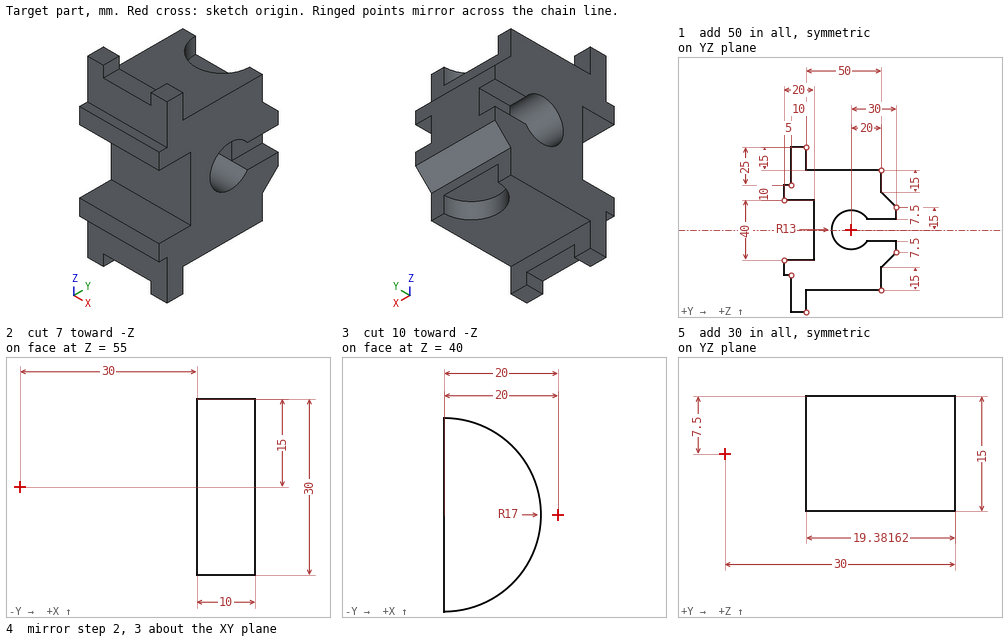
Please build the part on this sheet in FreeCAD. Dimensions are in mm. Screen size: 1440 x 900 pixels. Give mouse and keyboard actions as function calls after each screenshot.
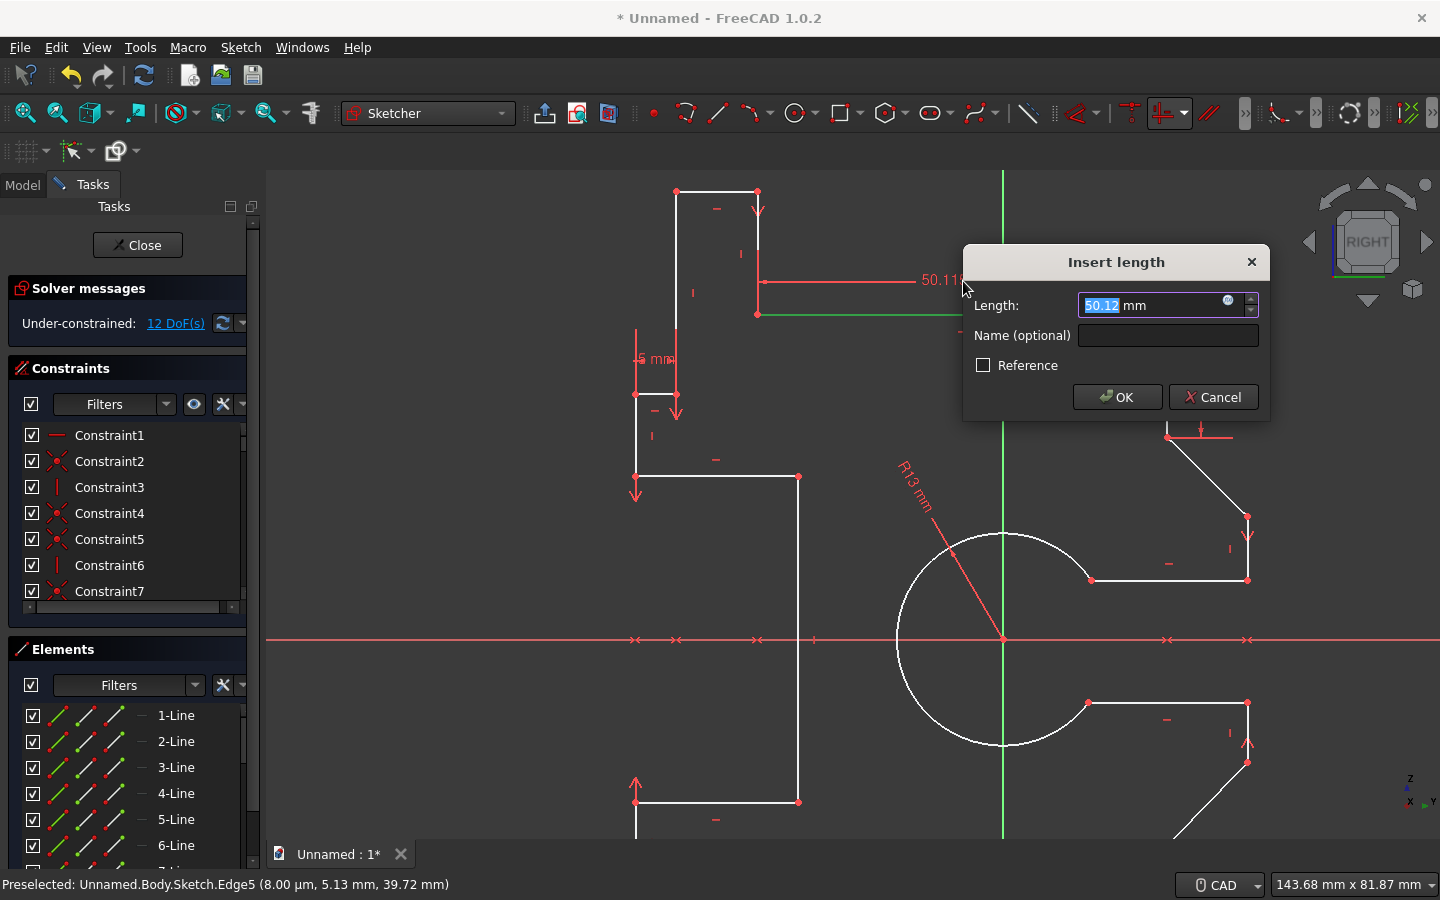
text(50)
key(Return)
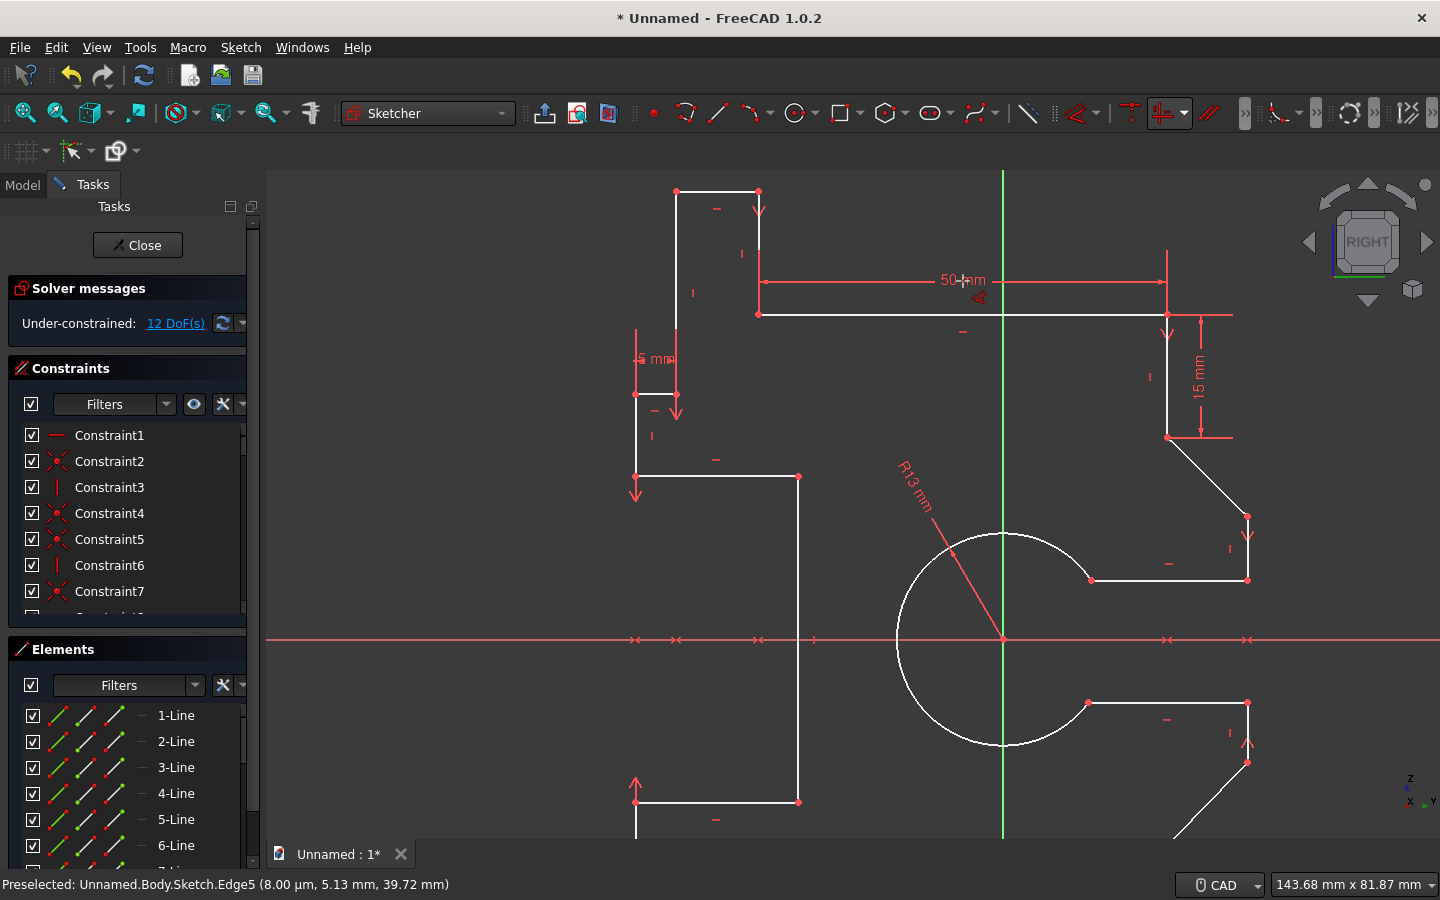
click(759, 278)
click(725, 256)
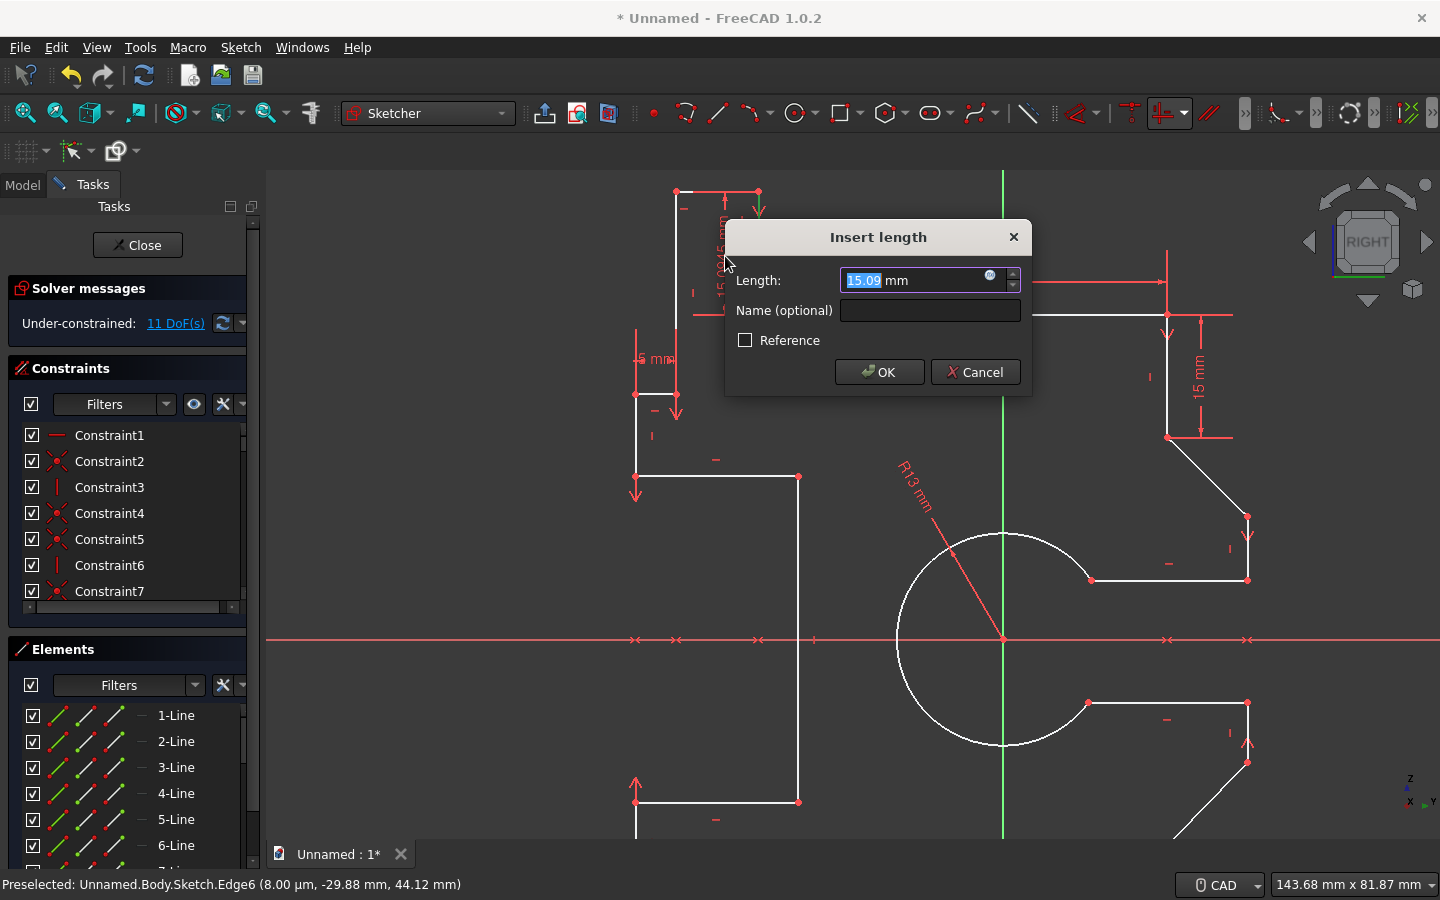
text(15)
key(Return)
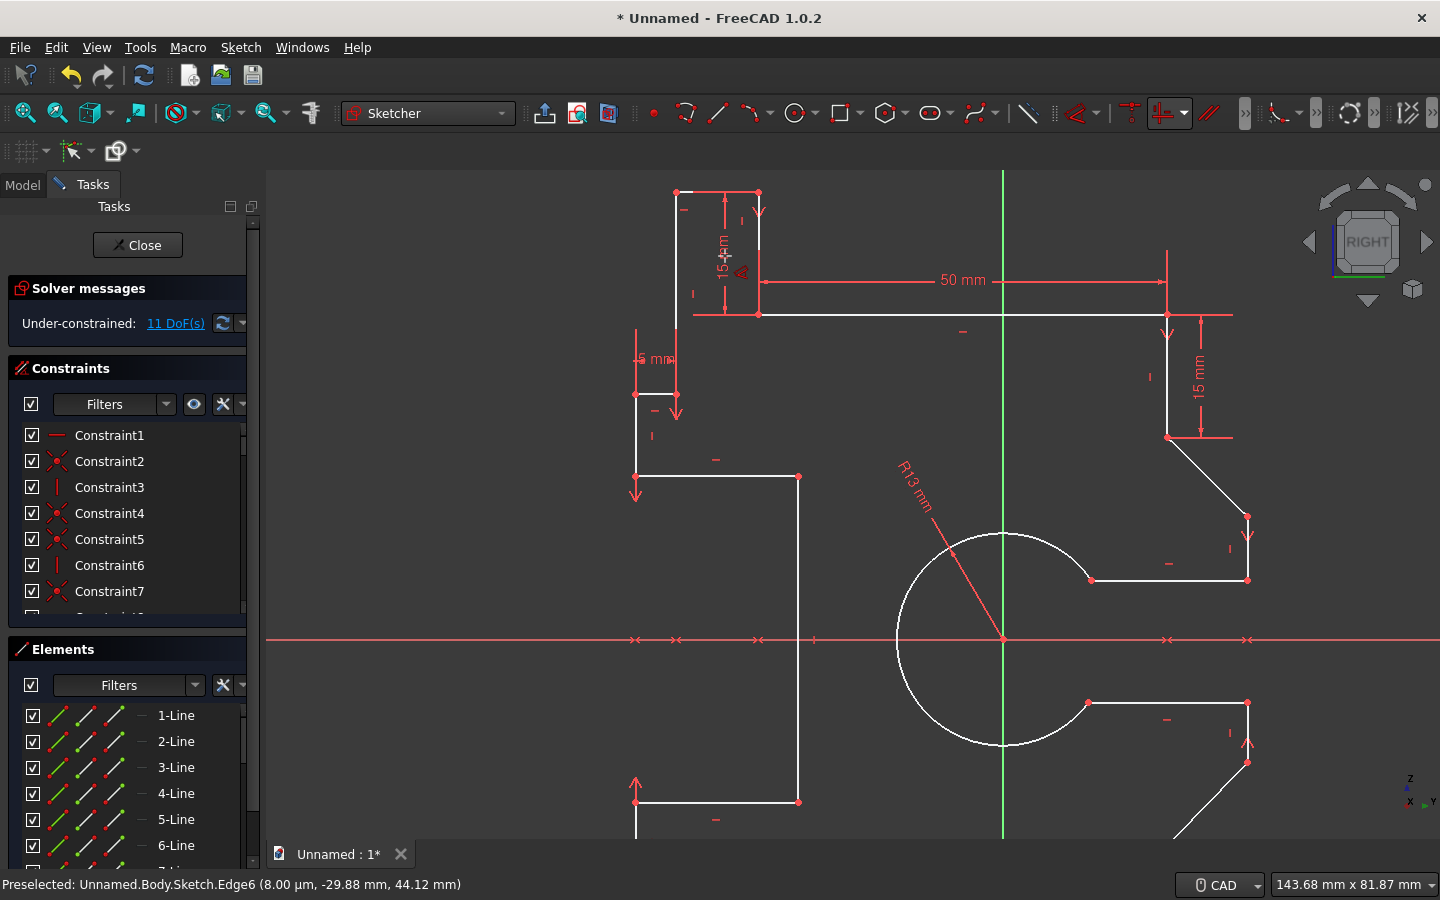
scroll(656, 394, down, 4)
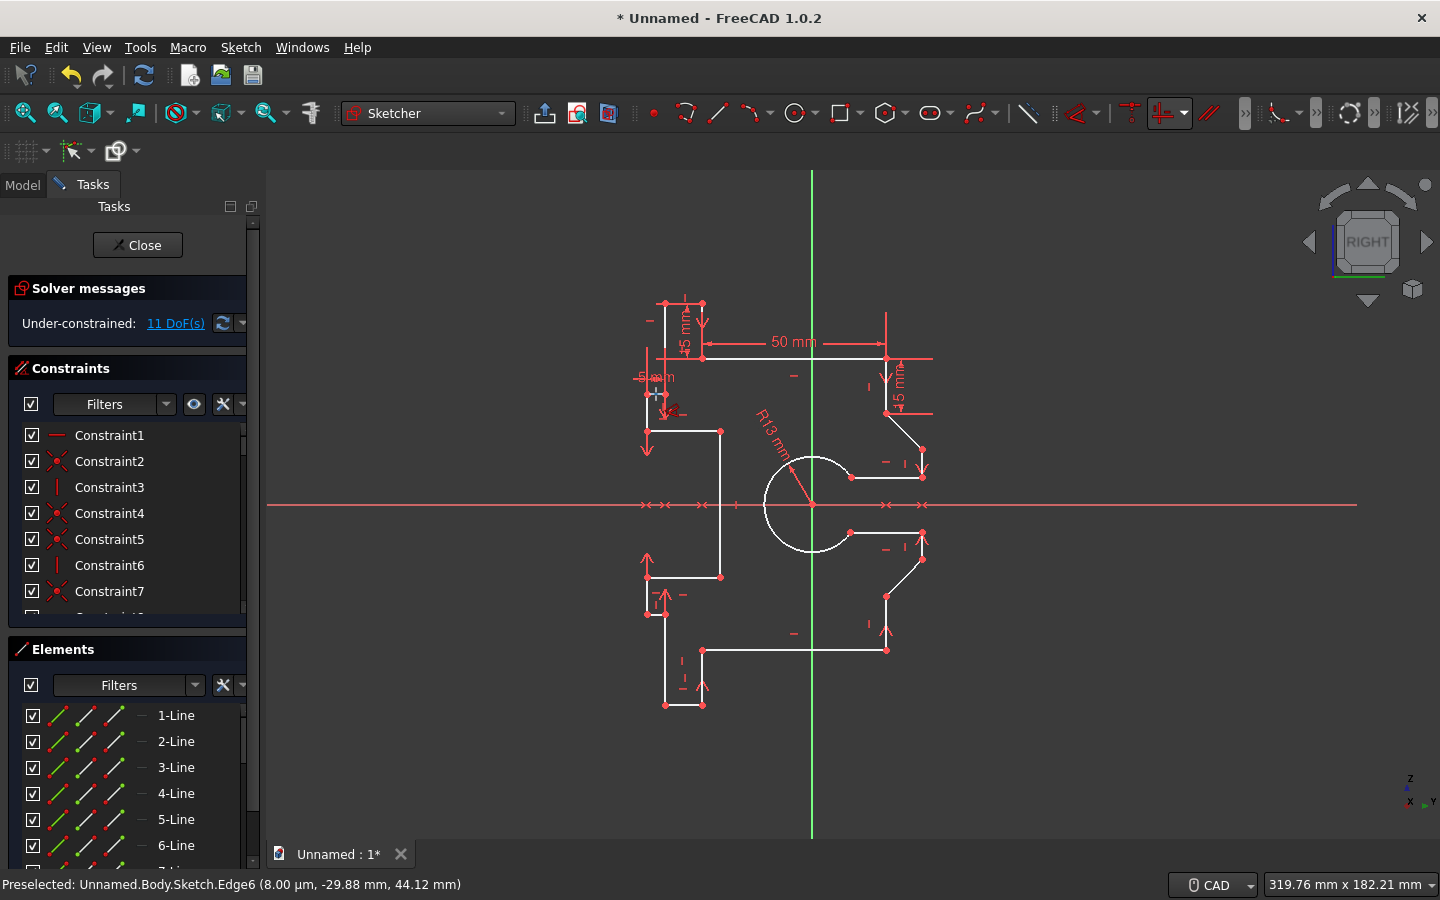
scroll(691, 304, up, 2)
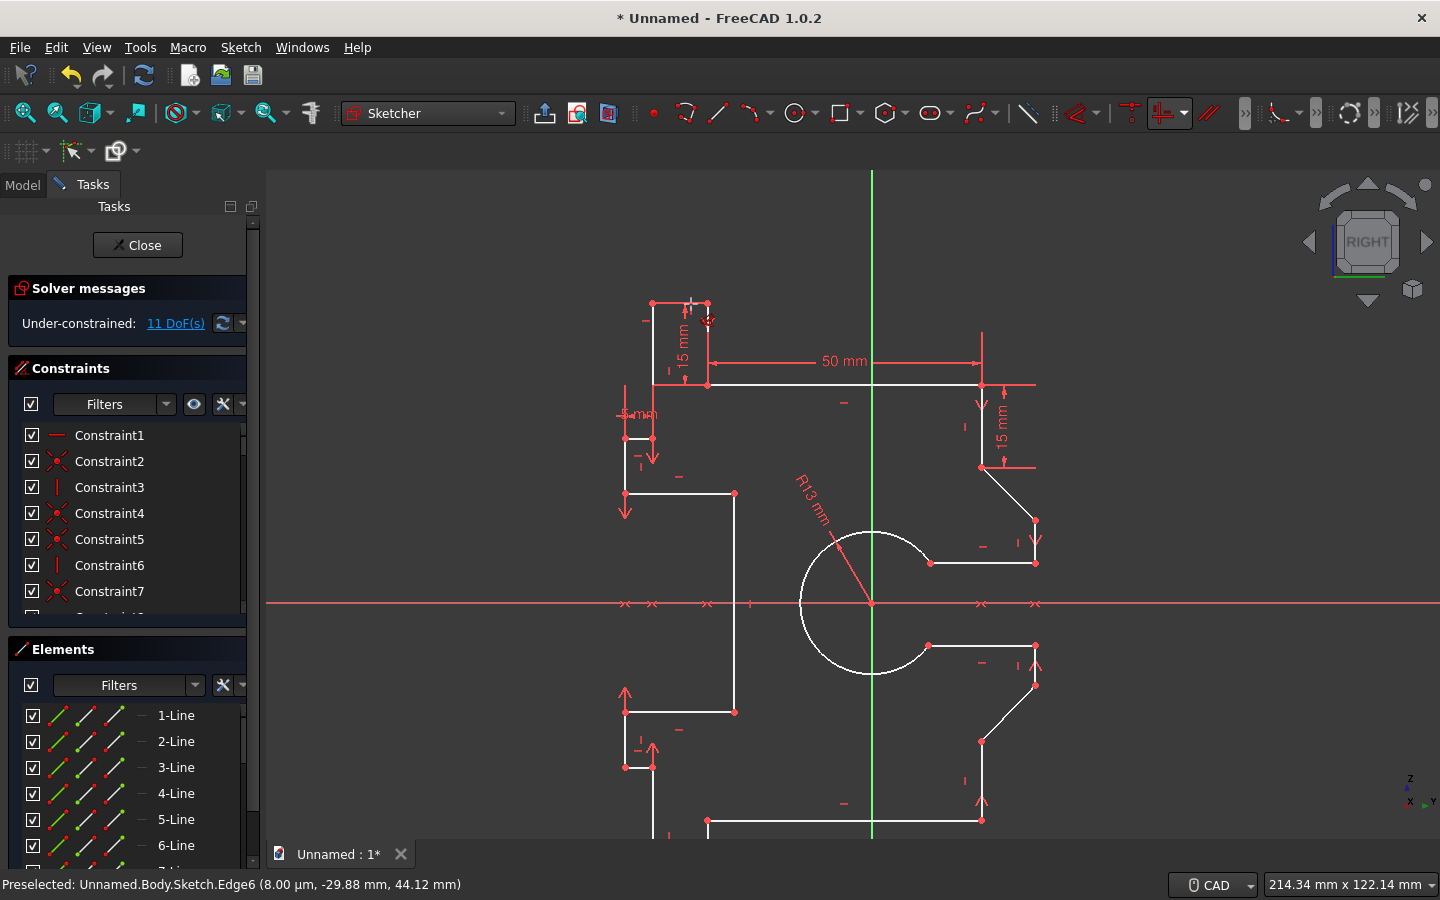
click(691, 303)
click(680, 269)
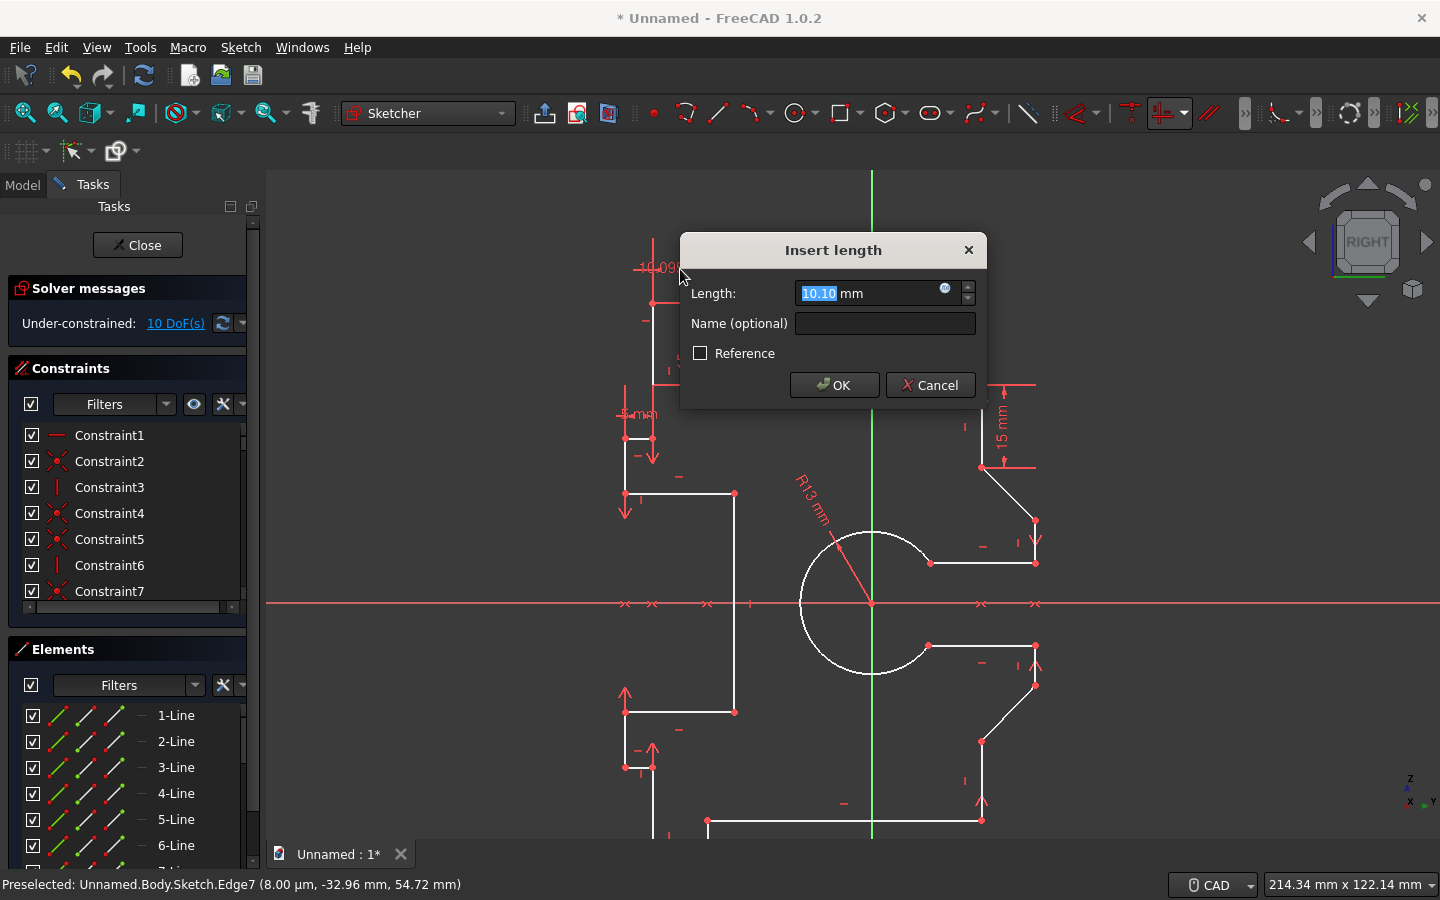
text(10)
key(Return)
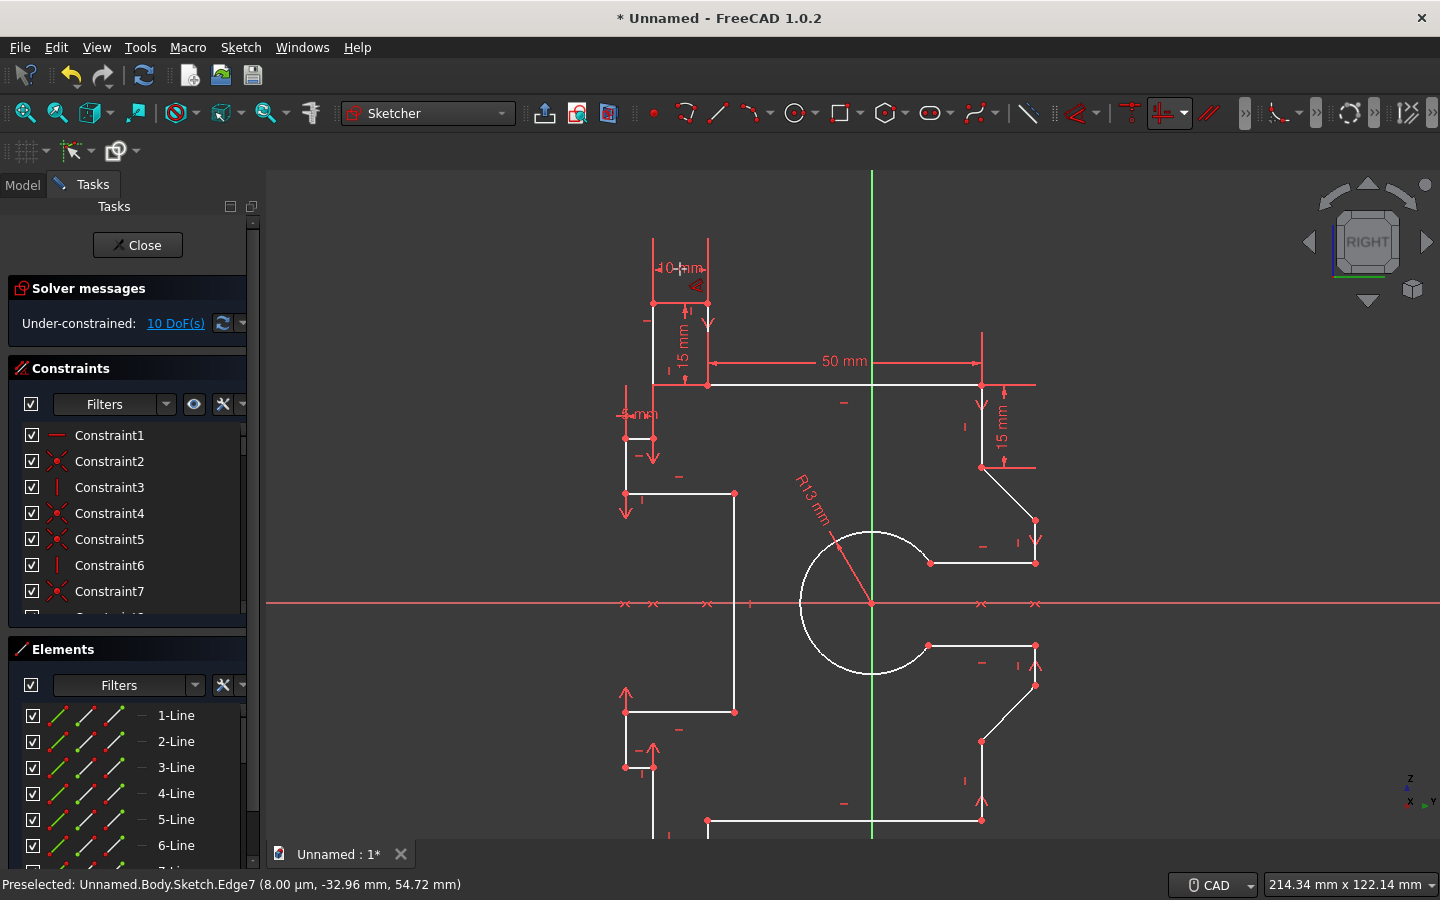
click(653, 344)
click(619, 371)